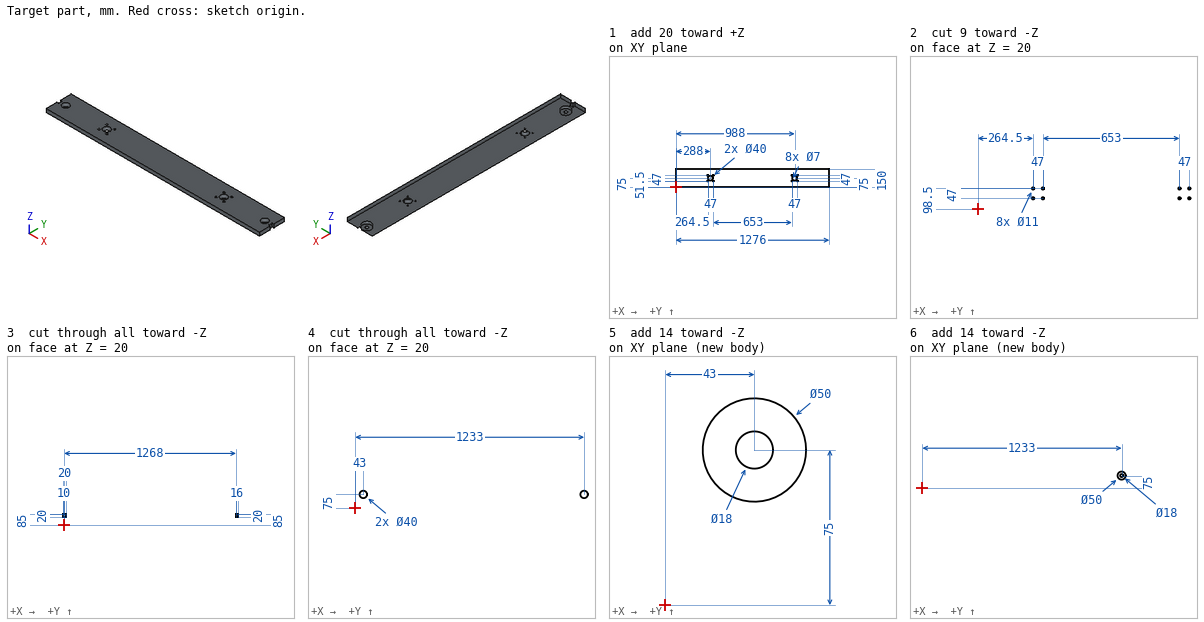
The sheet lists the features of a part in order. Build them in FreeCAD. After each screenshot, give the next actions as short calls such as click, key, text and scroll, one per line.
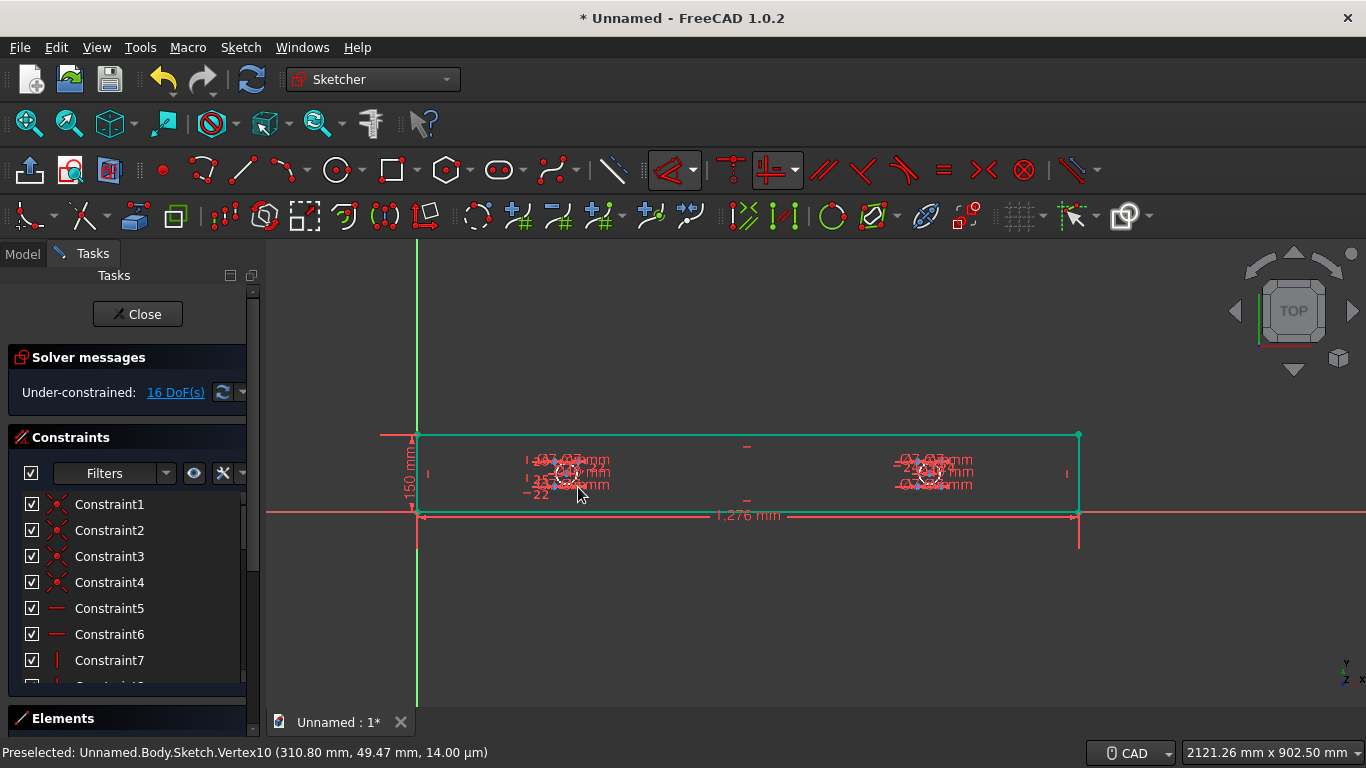
click(579, 462)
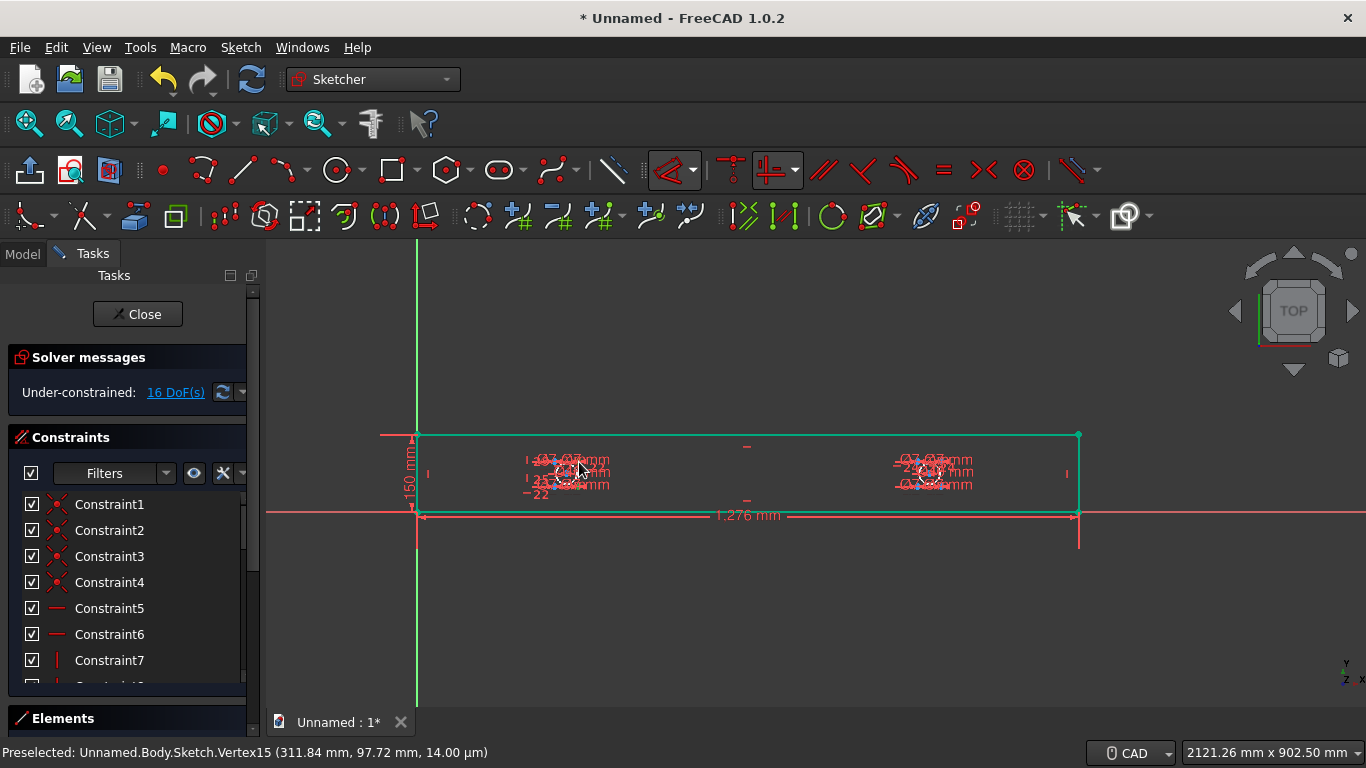
key(v)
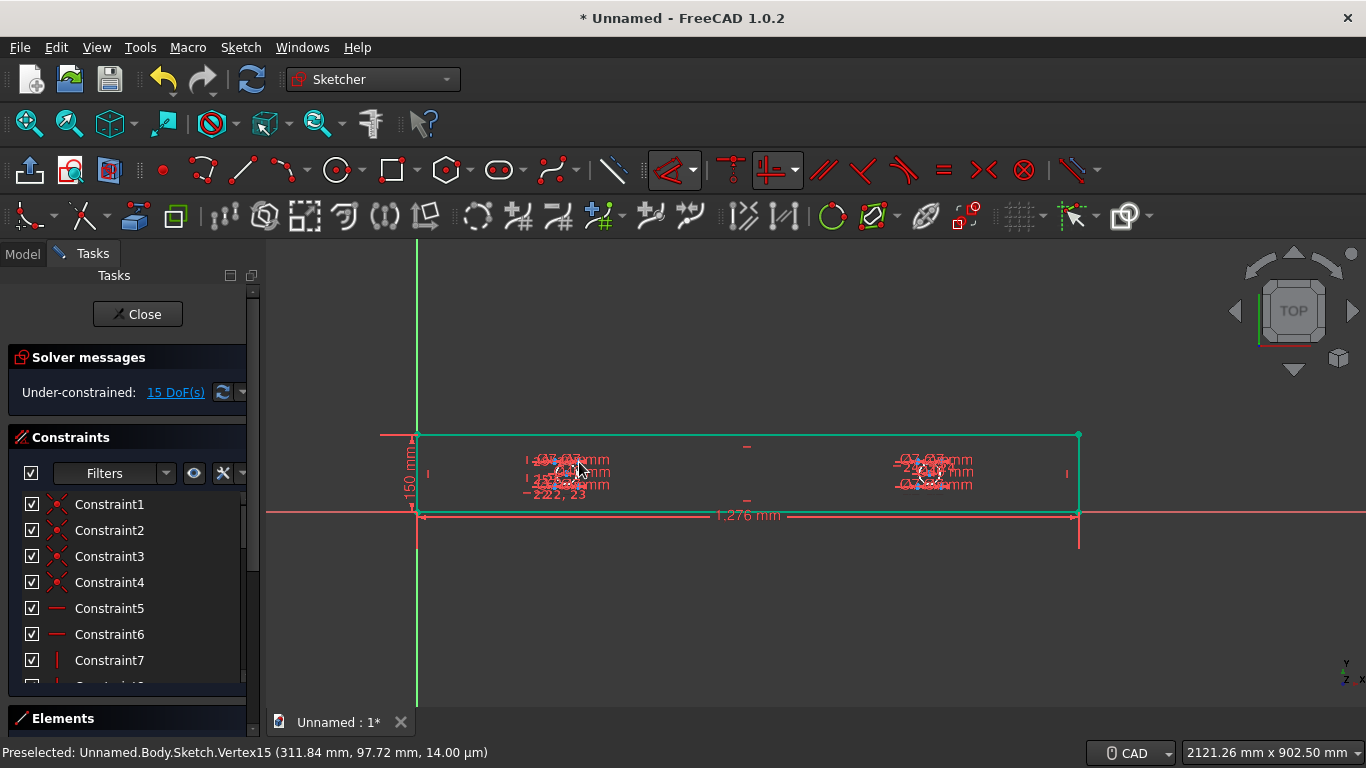
scroll(554, 462, up, 4)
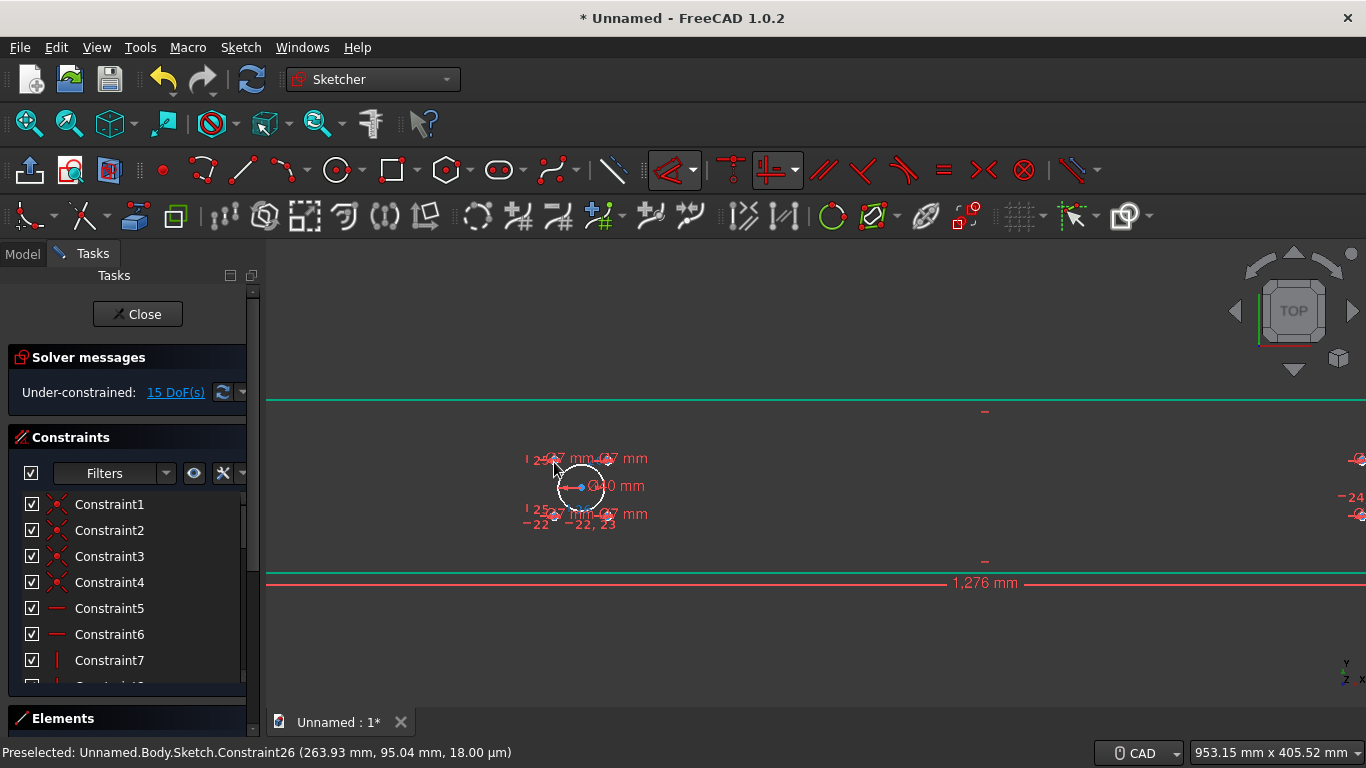
click(554, 460)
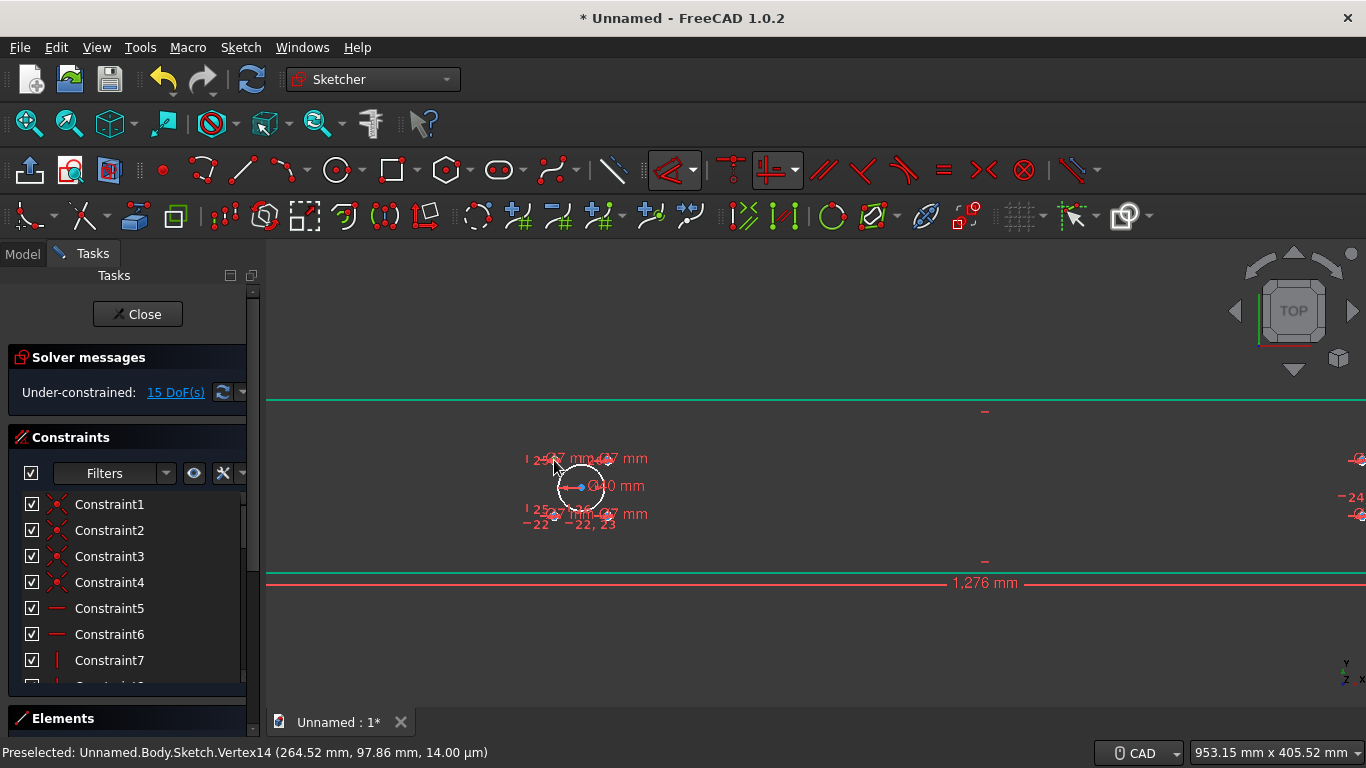
click(608, 461)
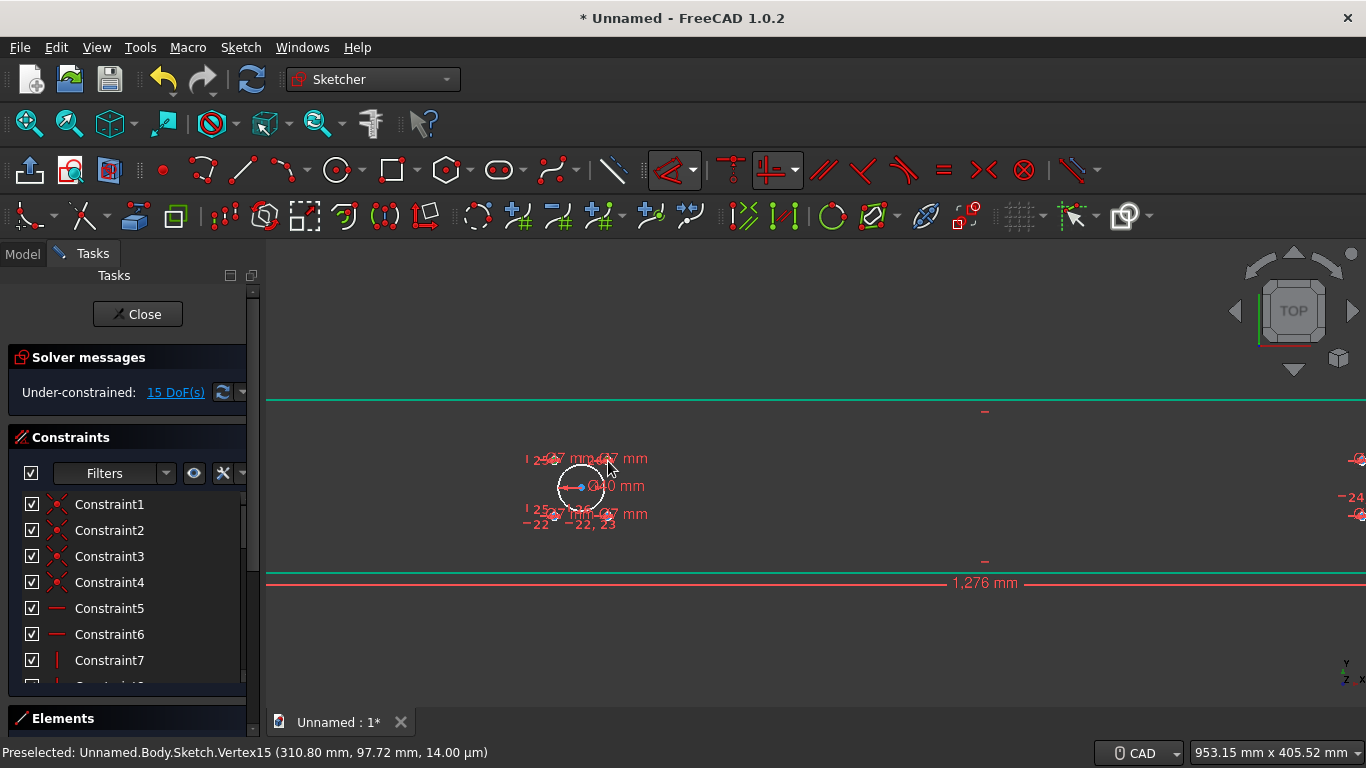
key(h)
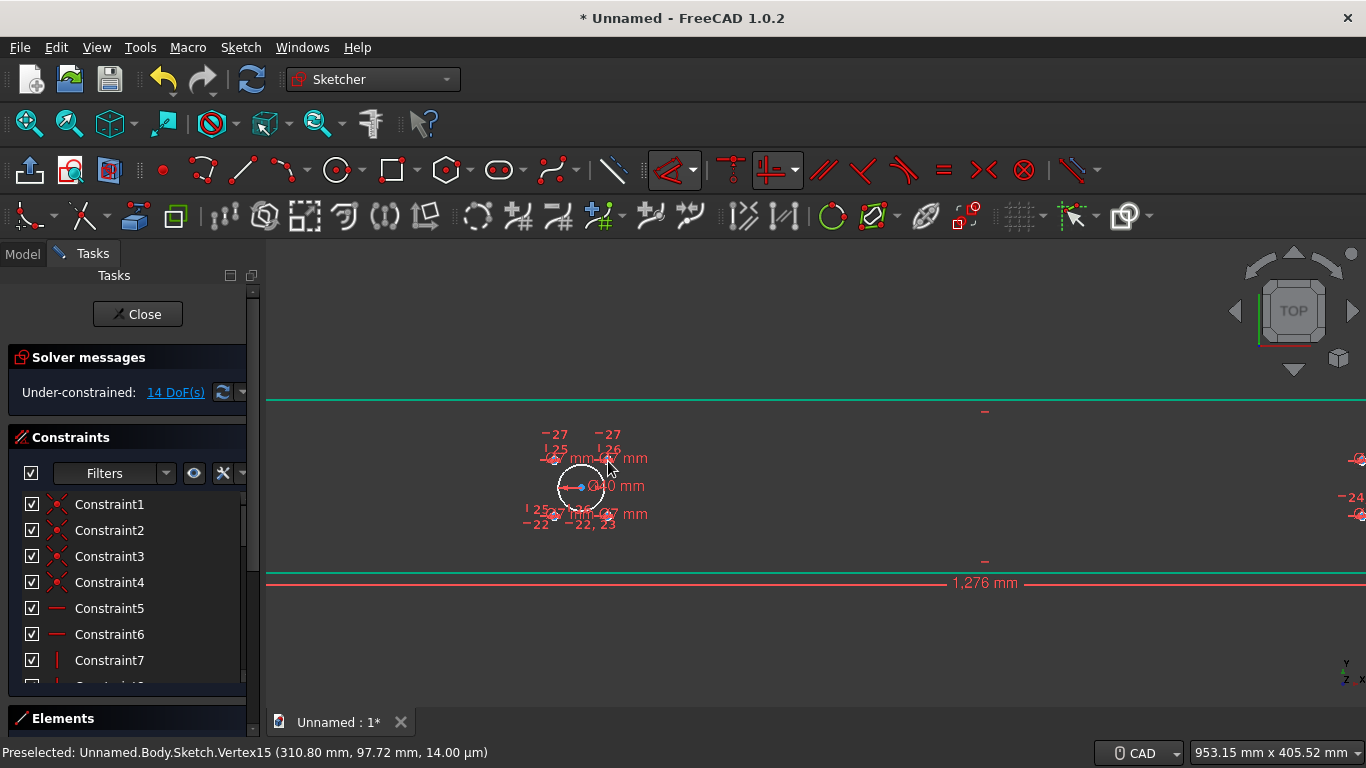
scroll(553, 462, down, 4)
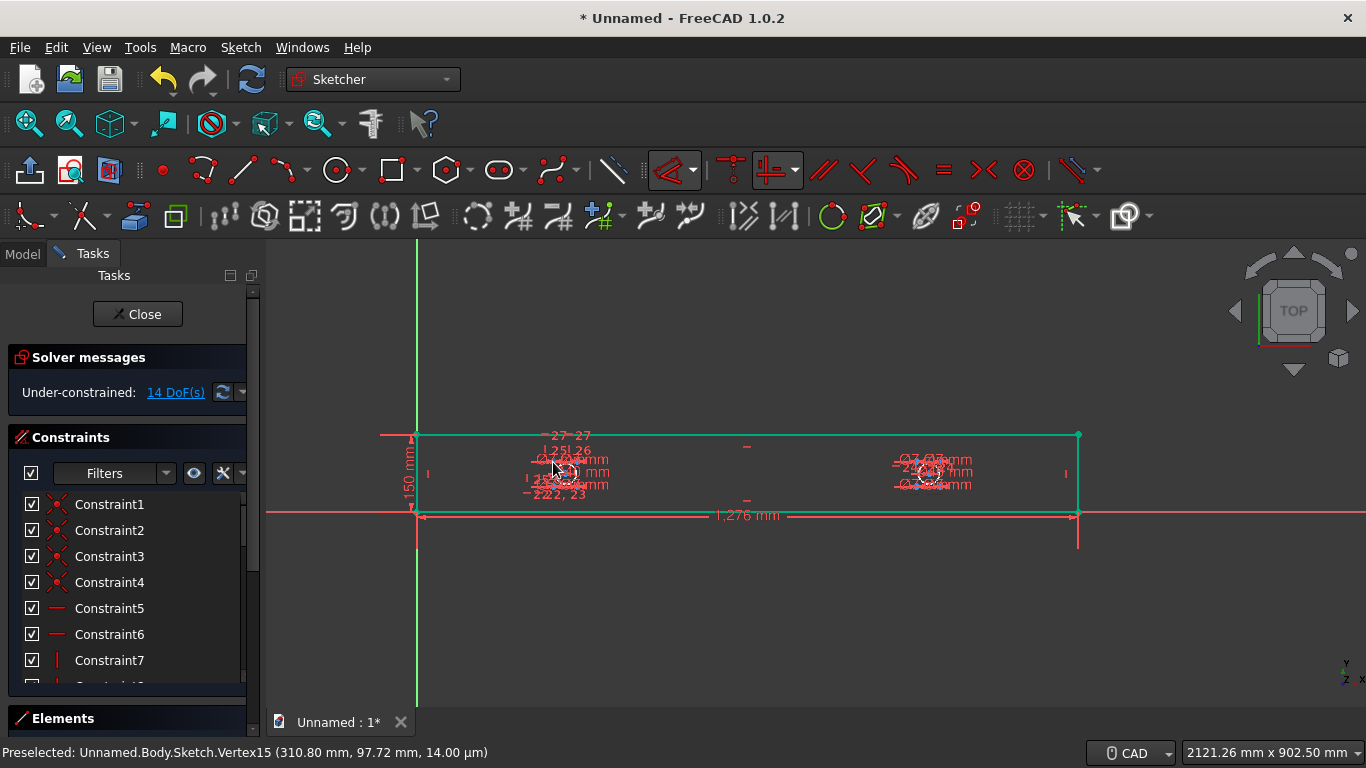
click(917, 487)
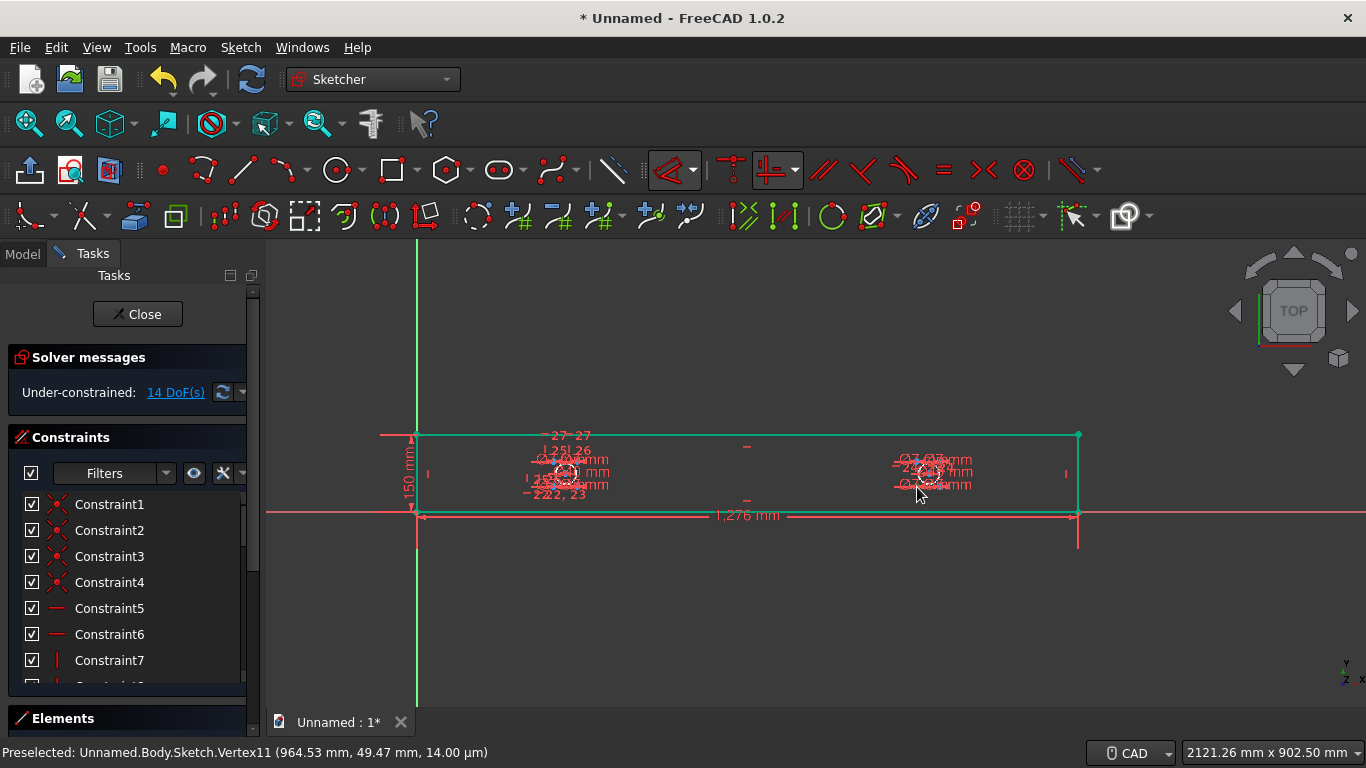
click(917, 462)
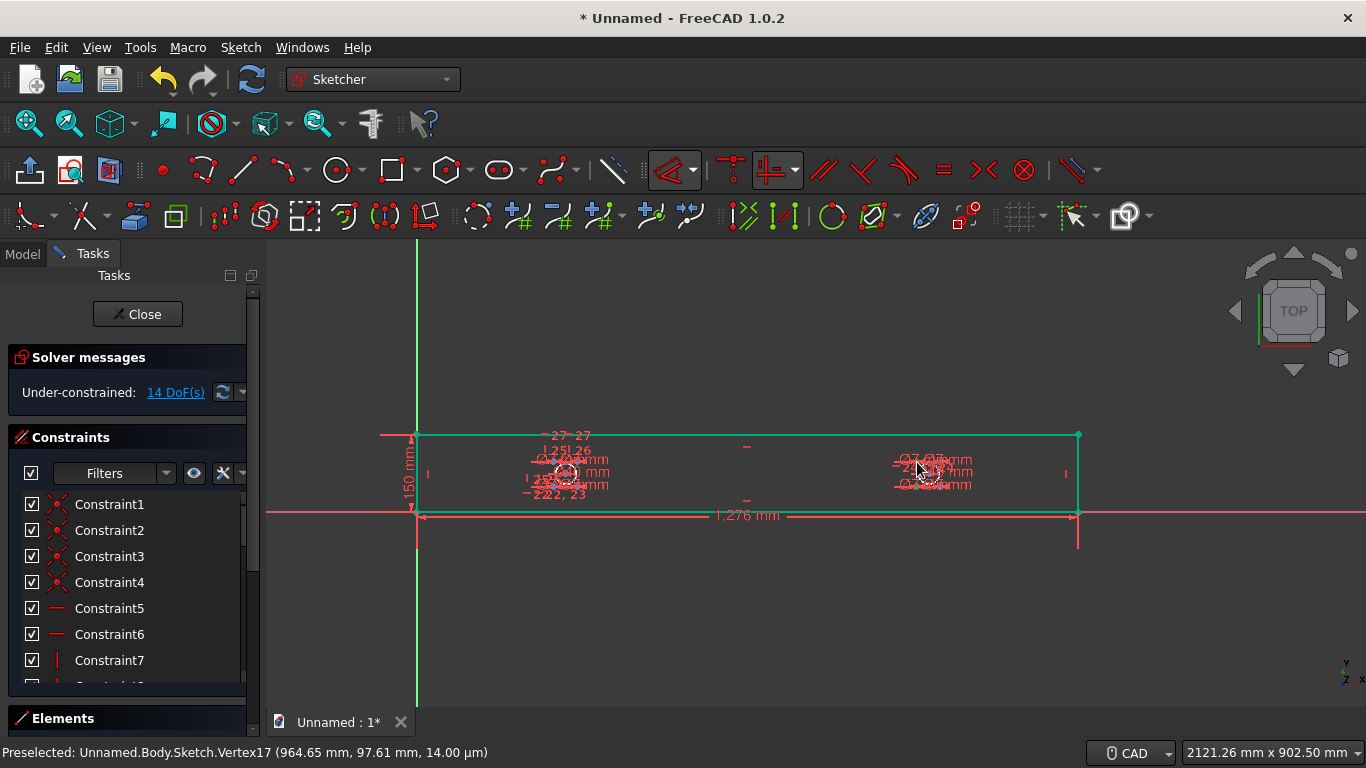
click(798, 170)